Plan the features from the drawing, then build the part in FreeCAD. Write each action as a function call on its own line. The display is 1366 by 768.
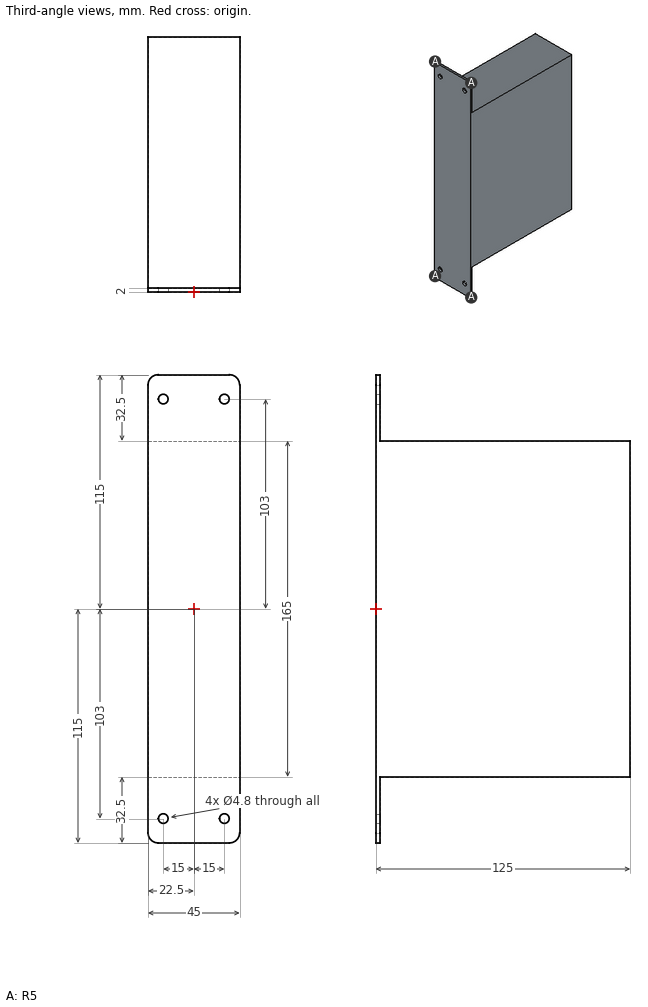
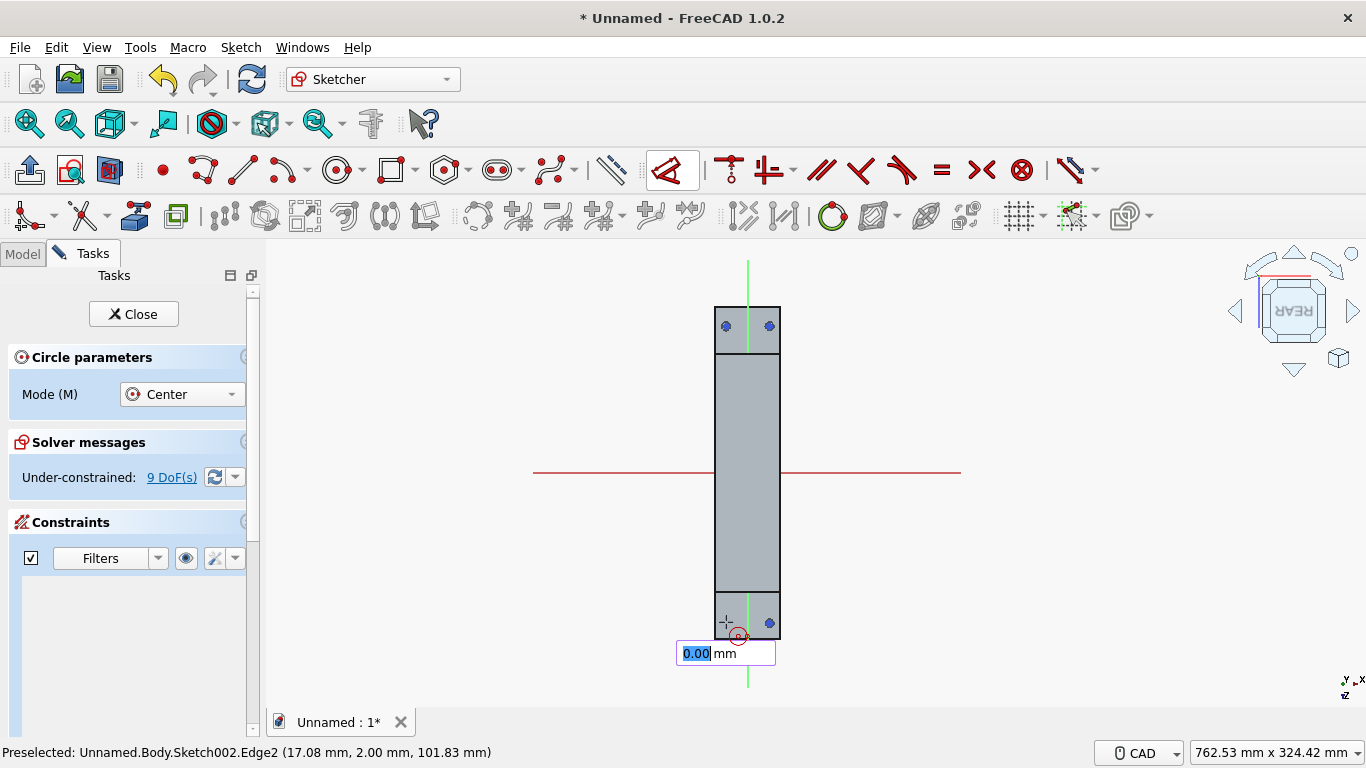
scroll(728, 619, up, 8)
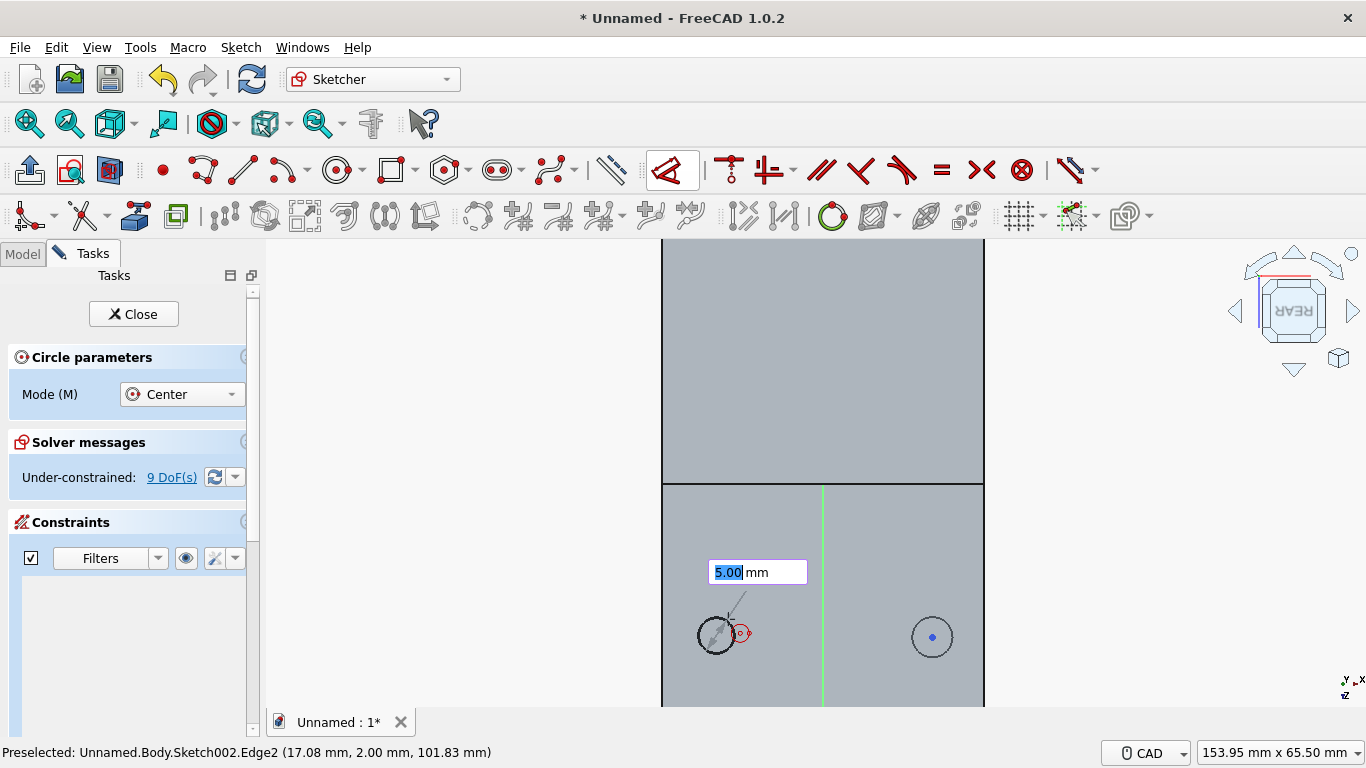
click(728, 618)
key(Escape)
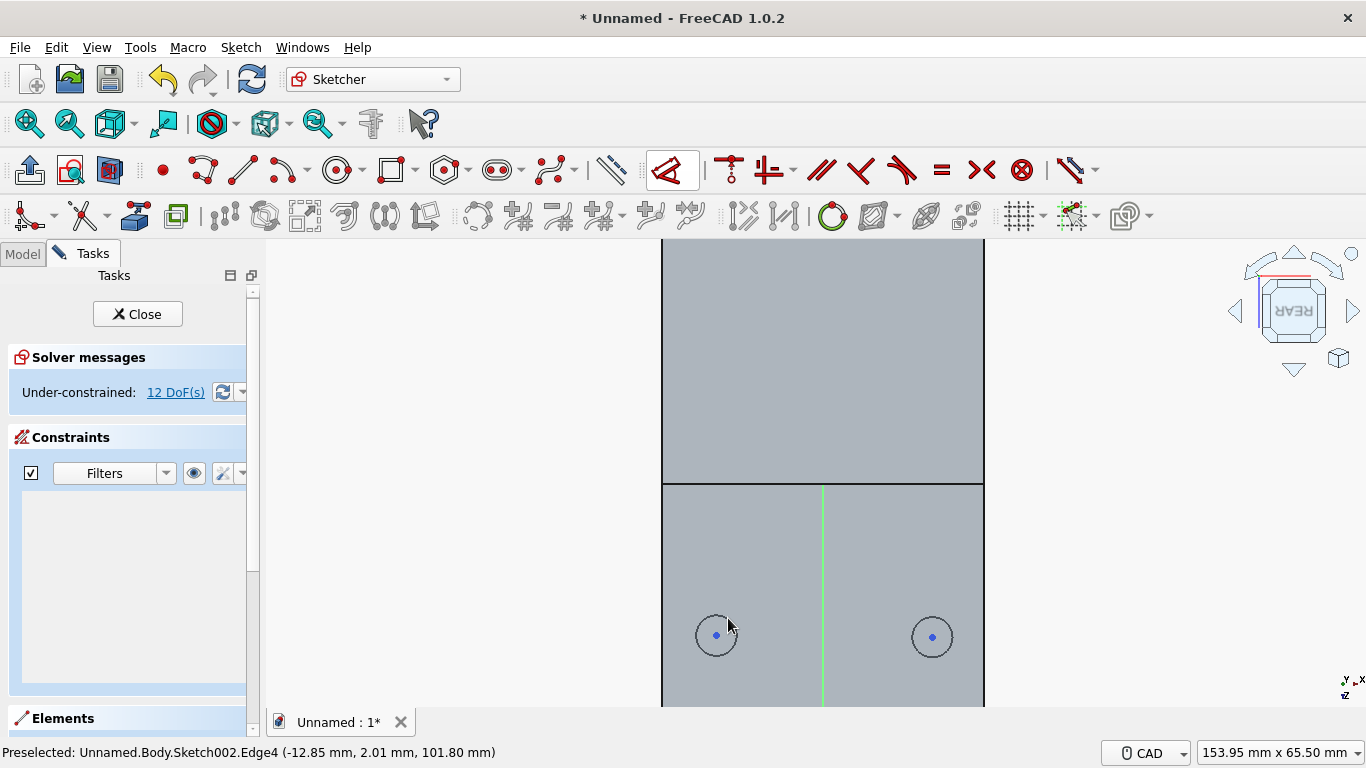
scroll(728, 619, down, 8)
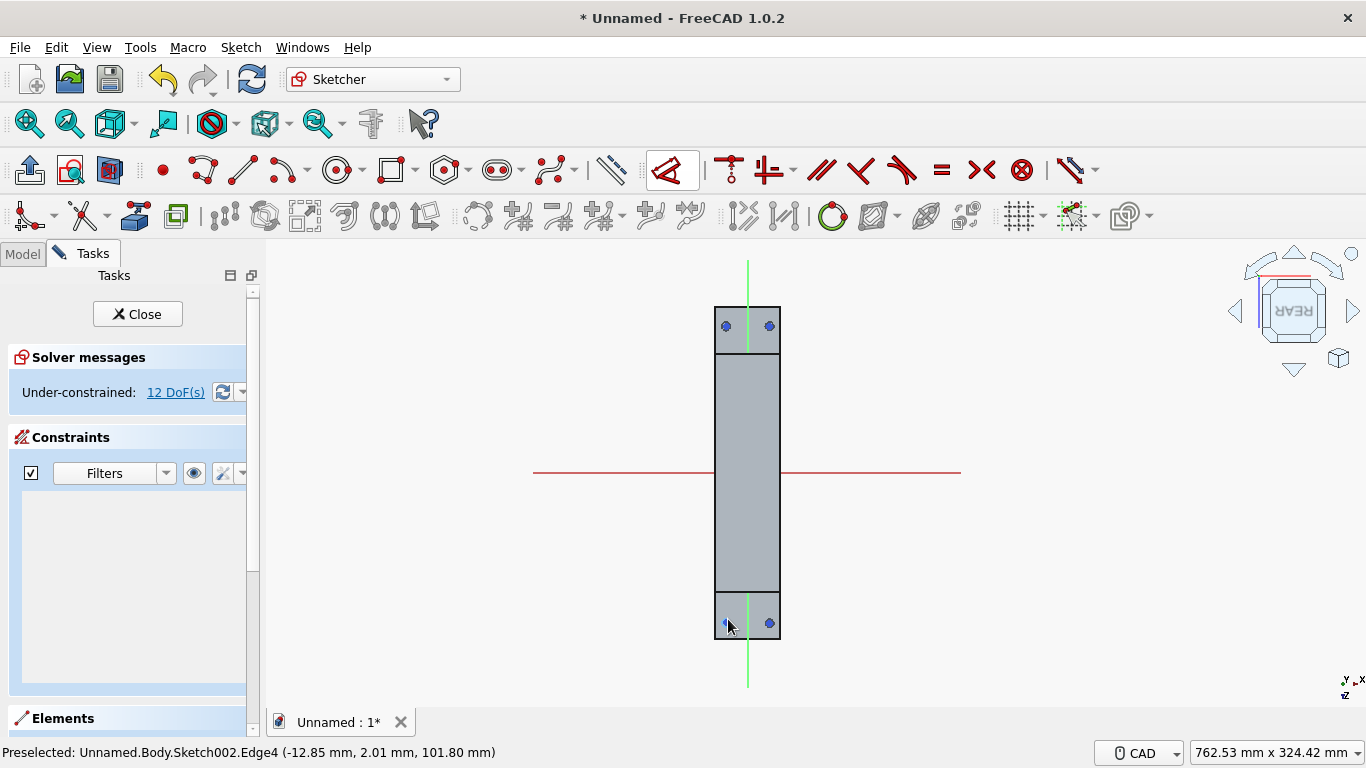
scroll(729, 323, up, 6)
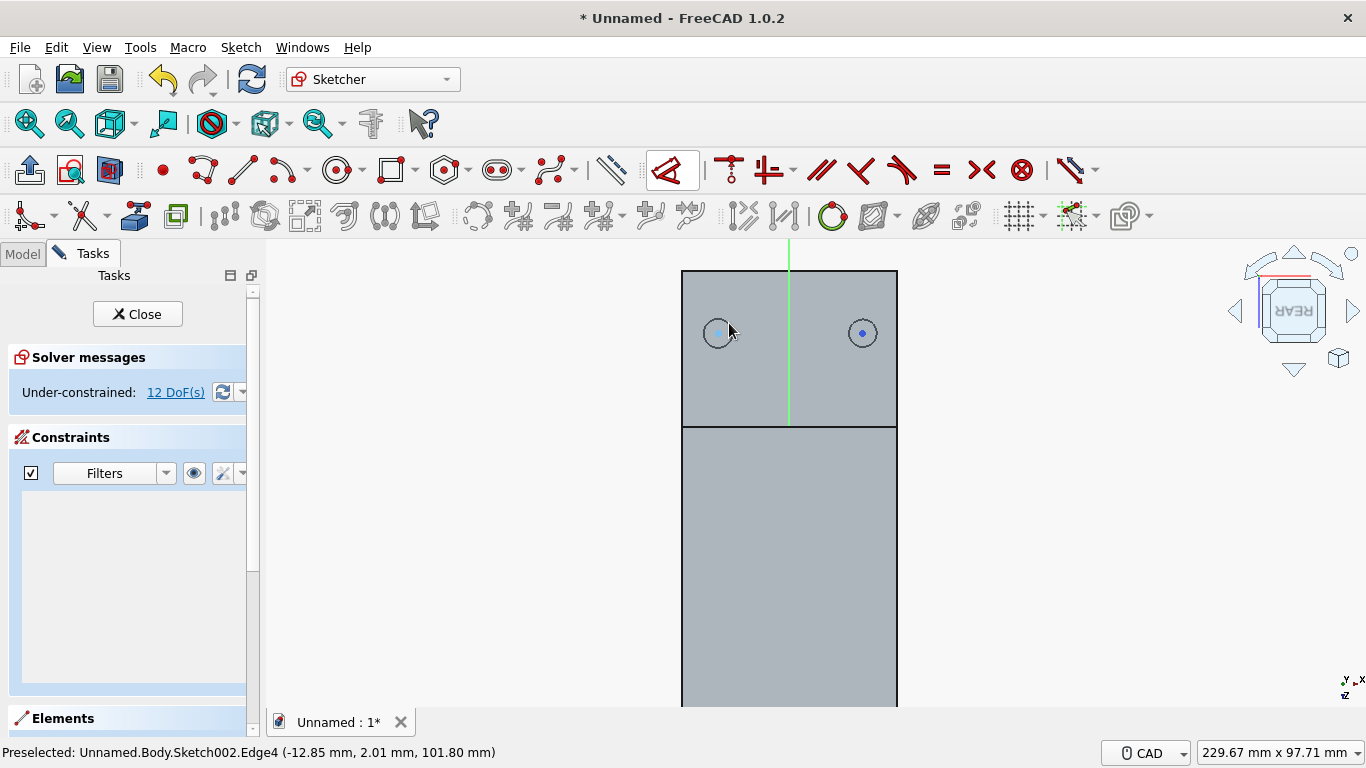
click(728, 323)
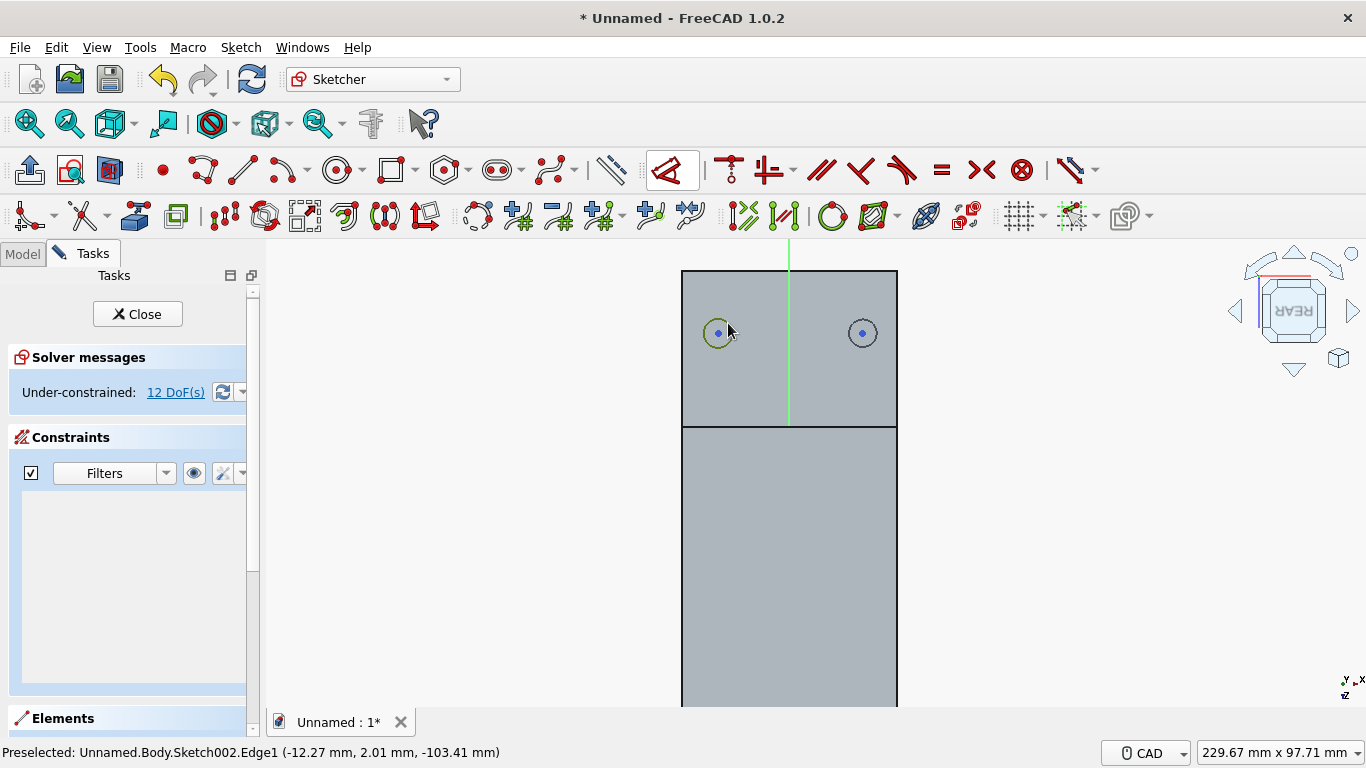
click(873, 323)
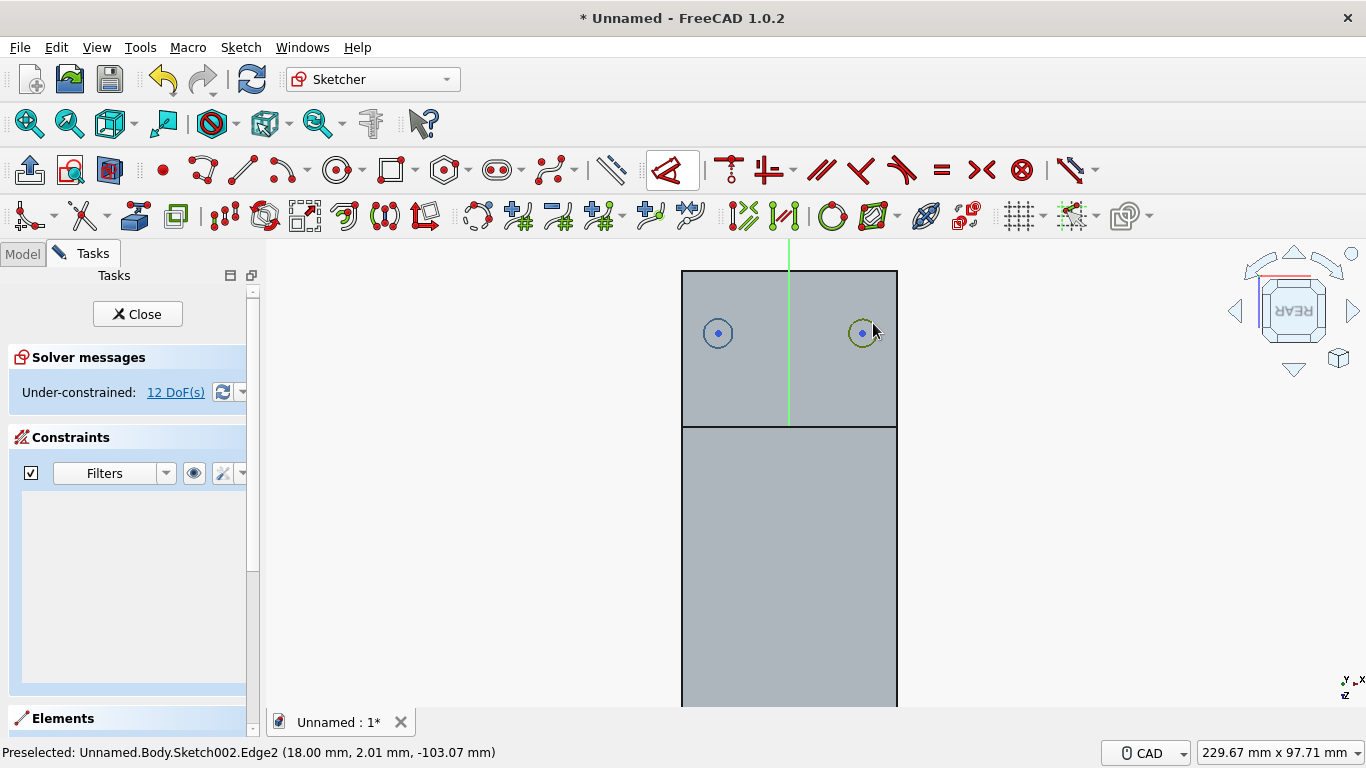
scroll(729, 323, down, 6)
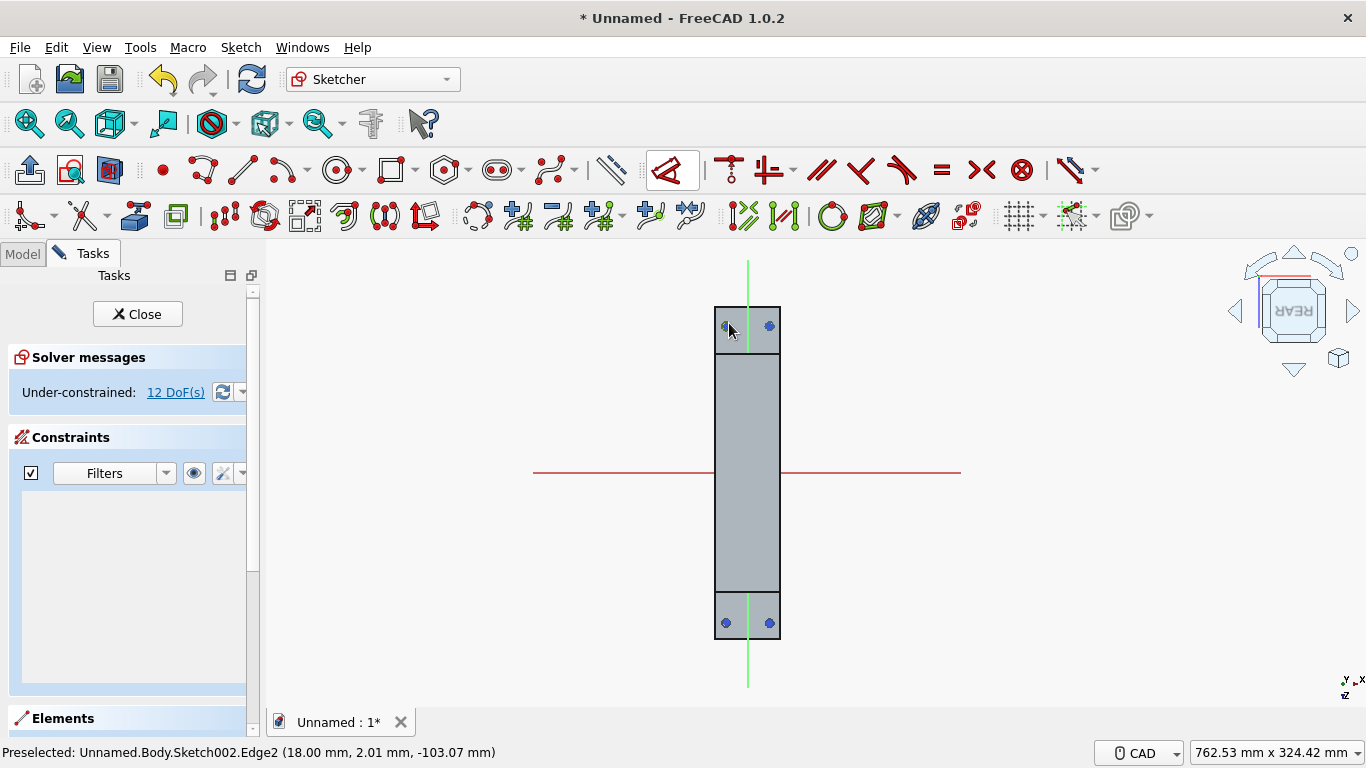
scroll(772, 620, up, 7)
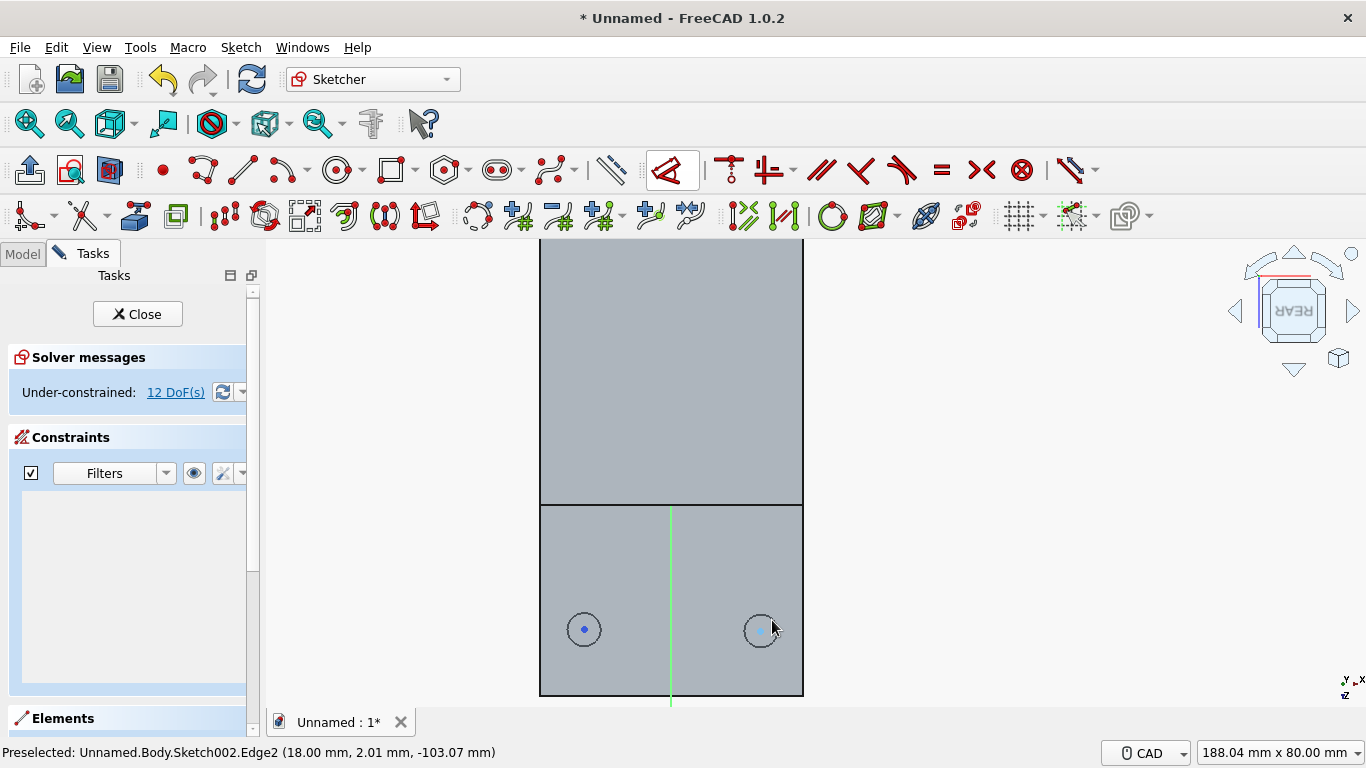
click(773, 619)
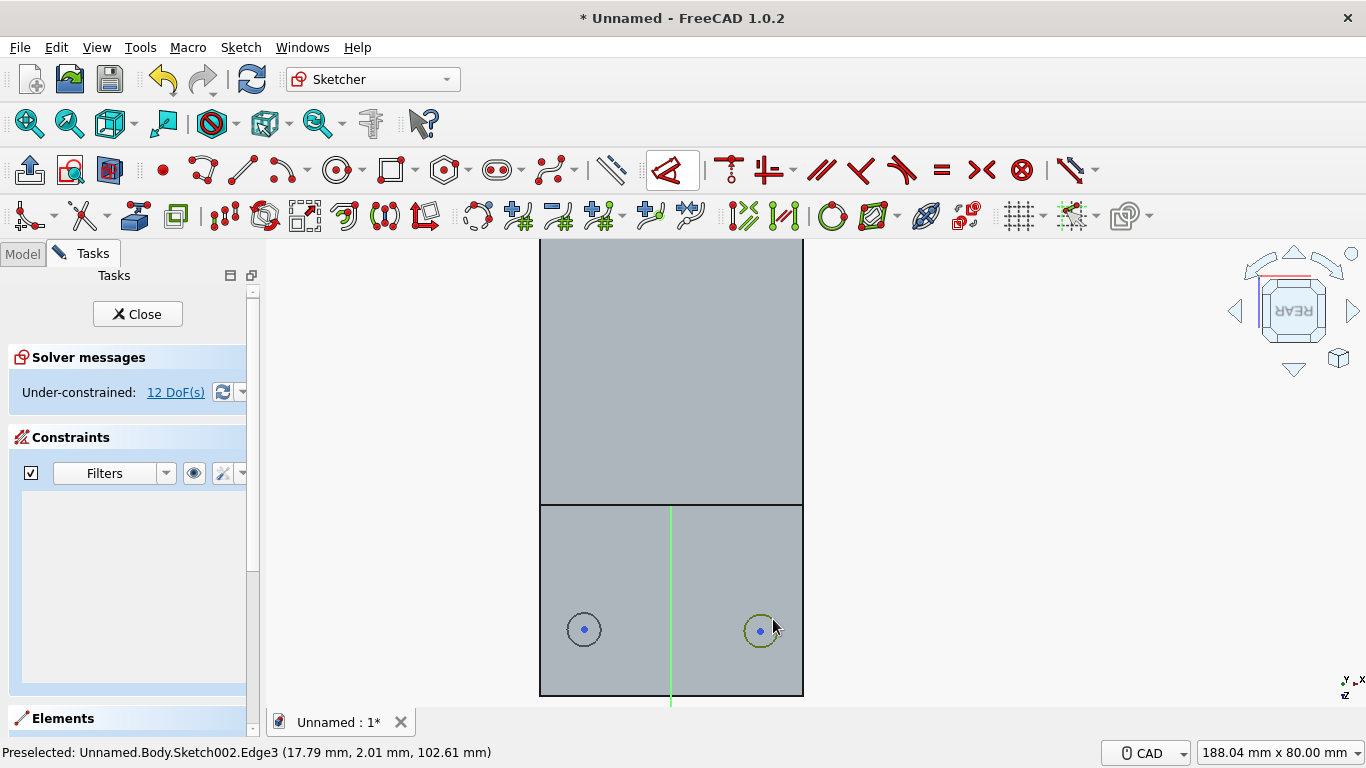
click(596, 618)